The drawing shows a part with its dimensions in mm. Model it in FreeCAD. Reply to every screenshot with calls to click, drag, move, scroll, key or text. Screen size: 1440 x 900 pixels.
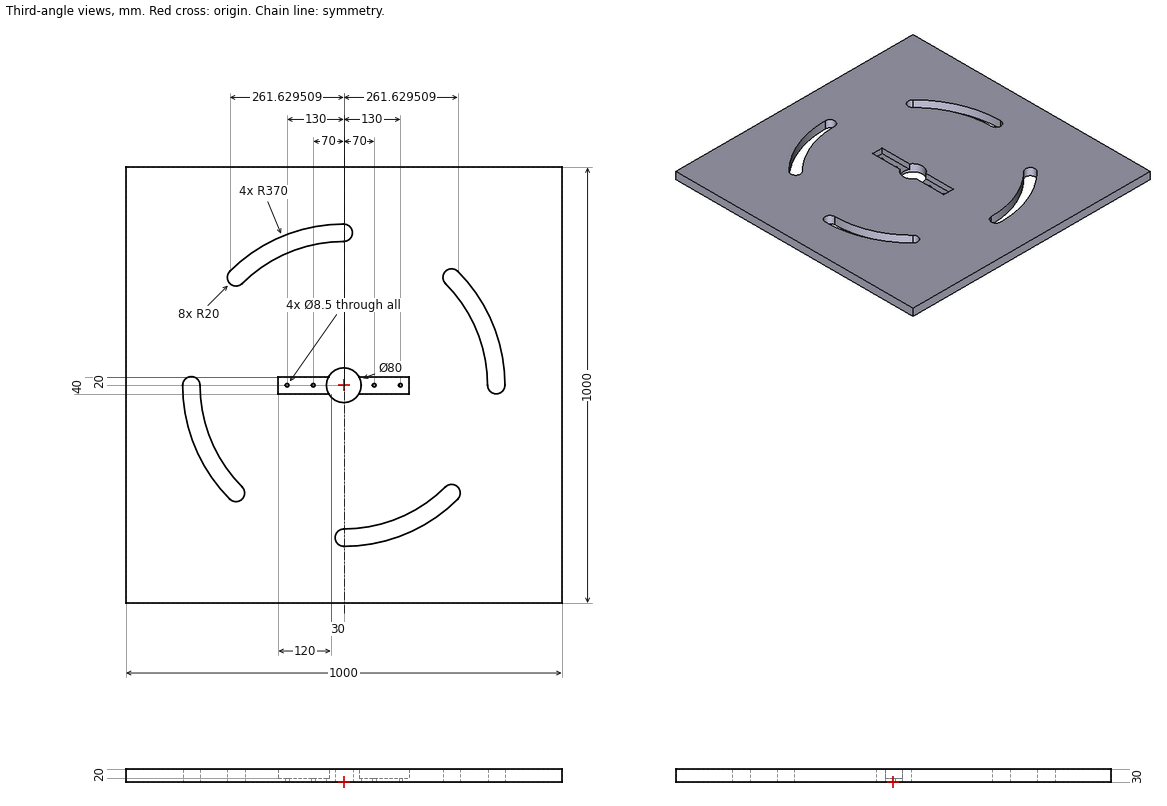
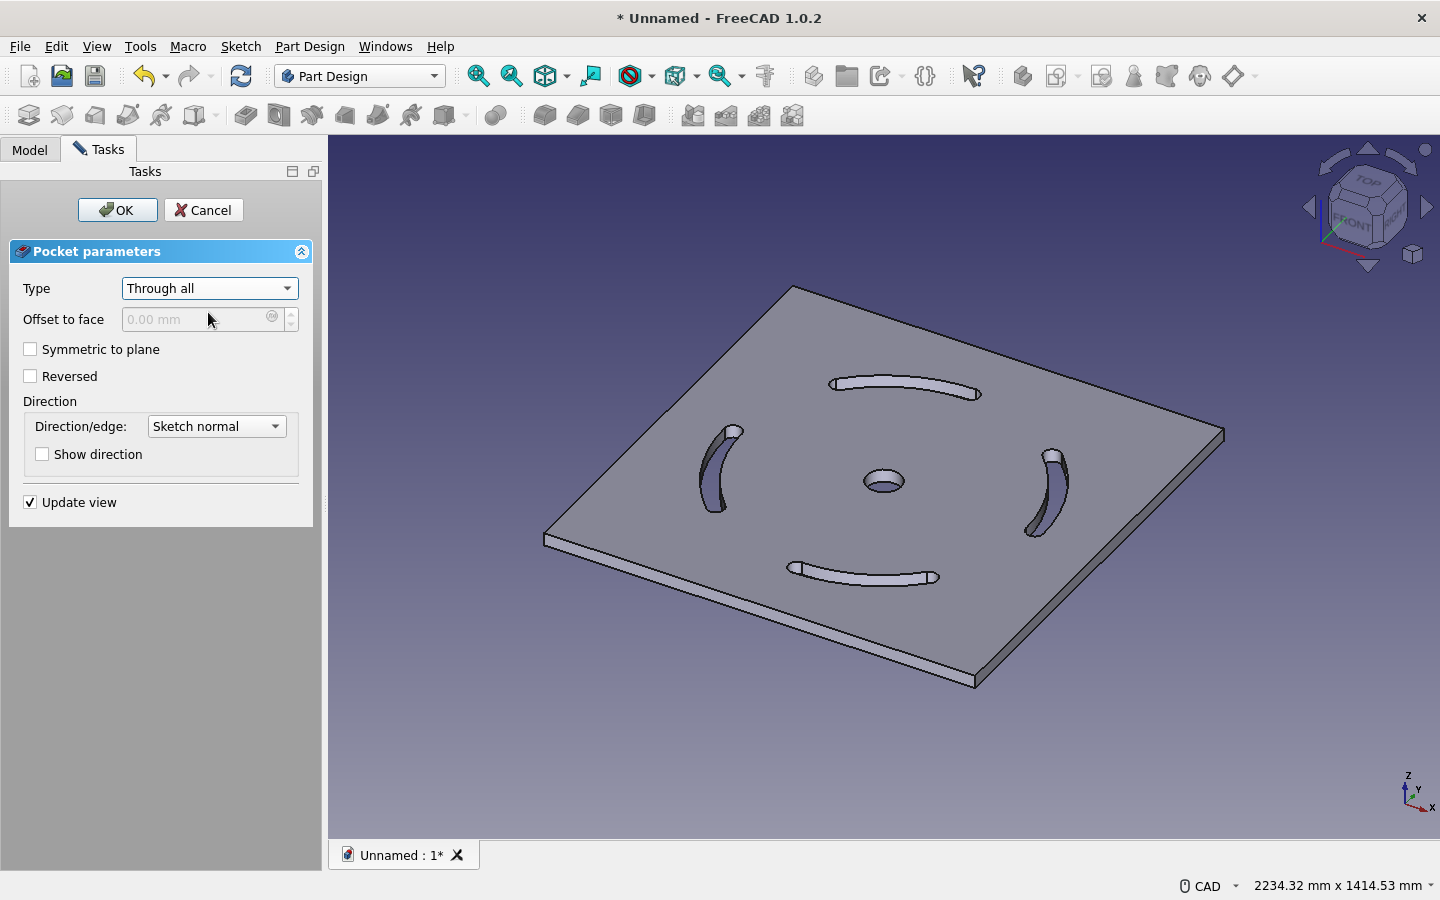
click(118, 210)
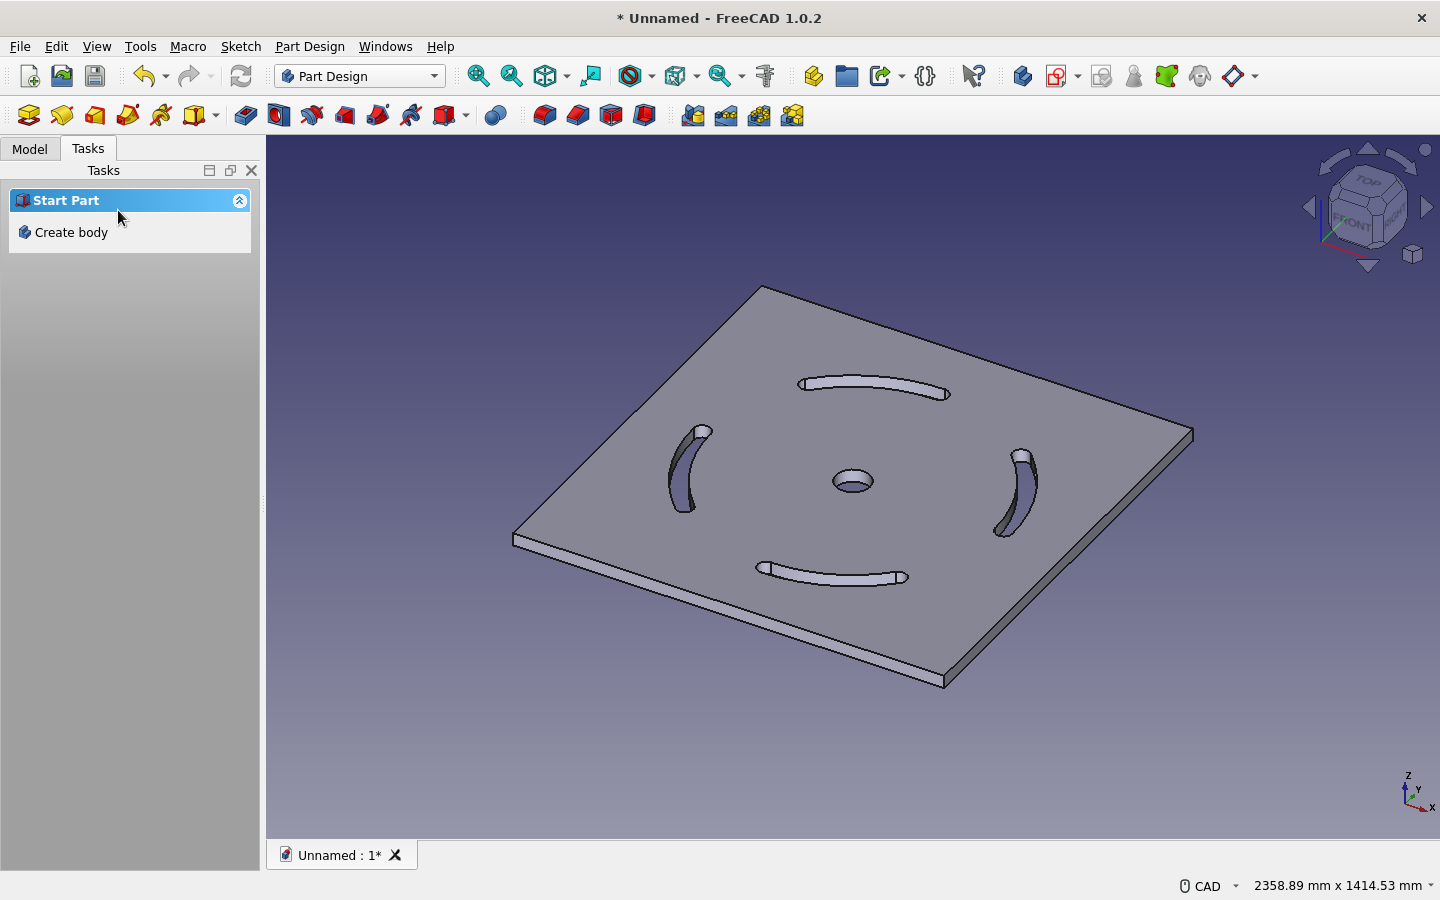
click(756, 495)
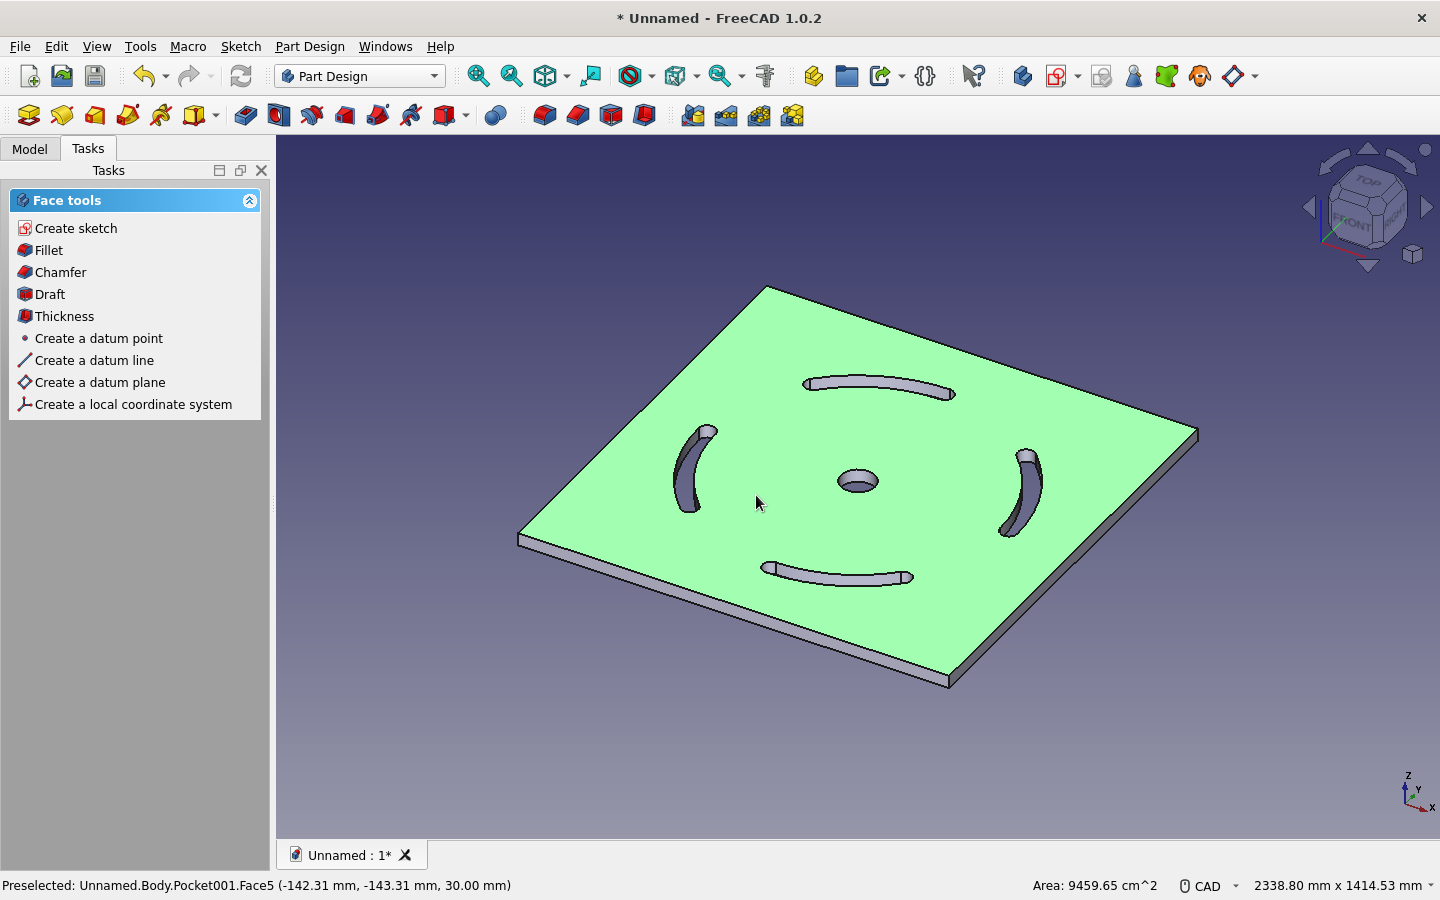
click(1056, 76)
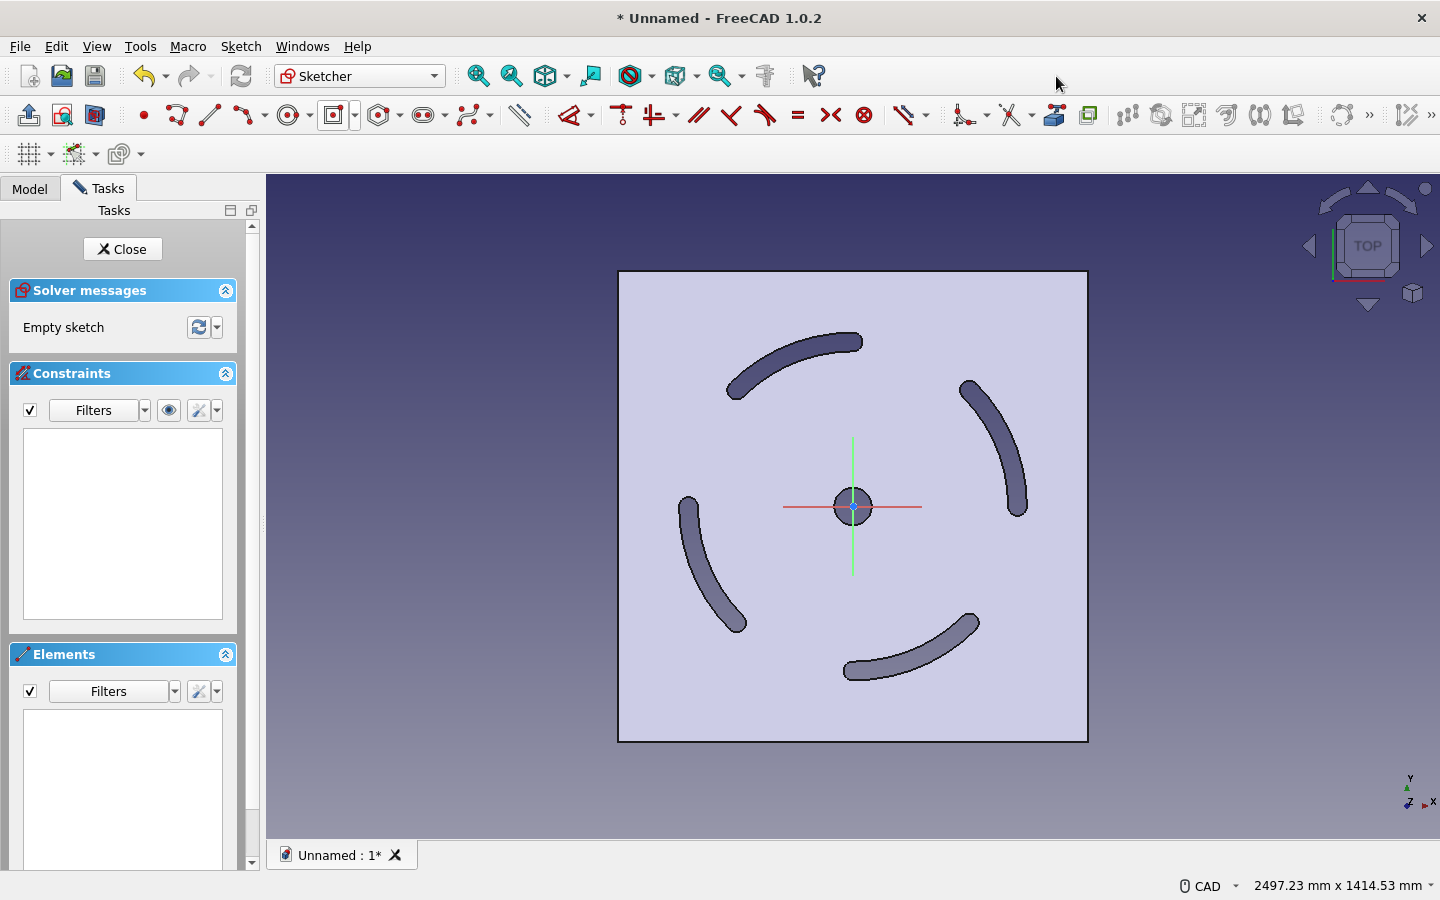
scroll(870, 506, up, 8)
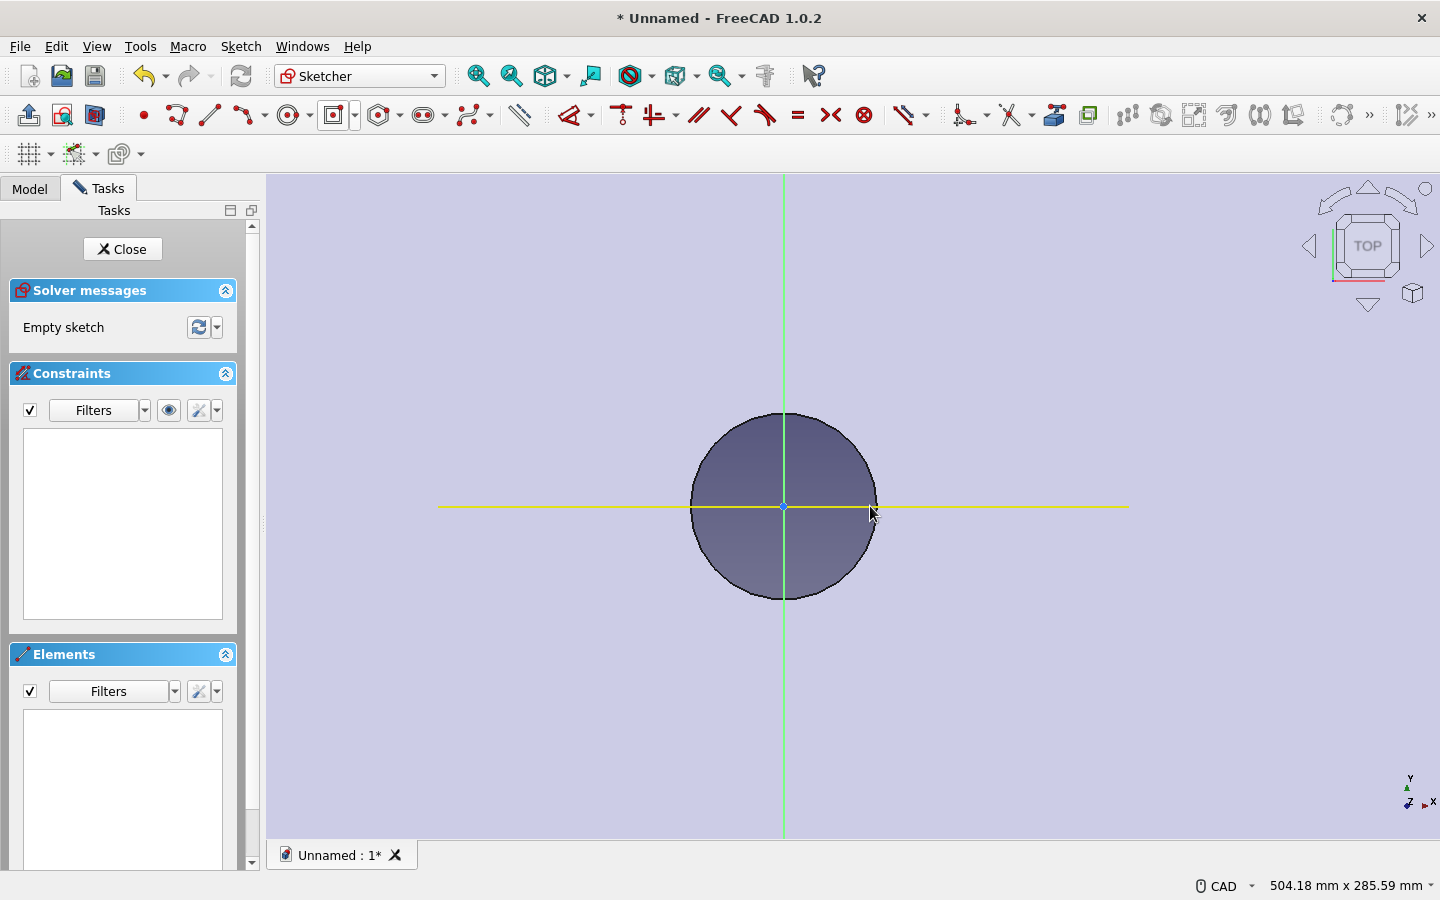
click(354, 116)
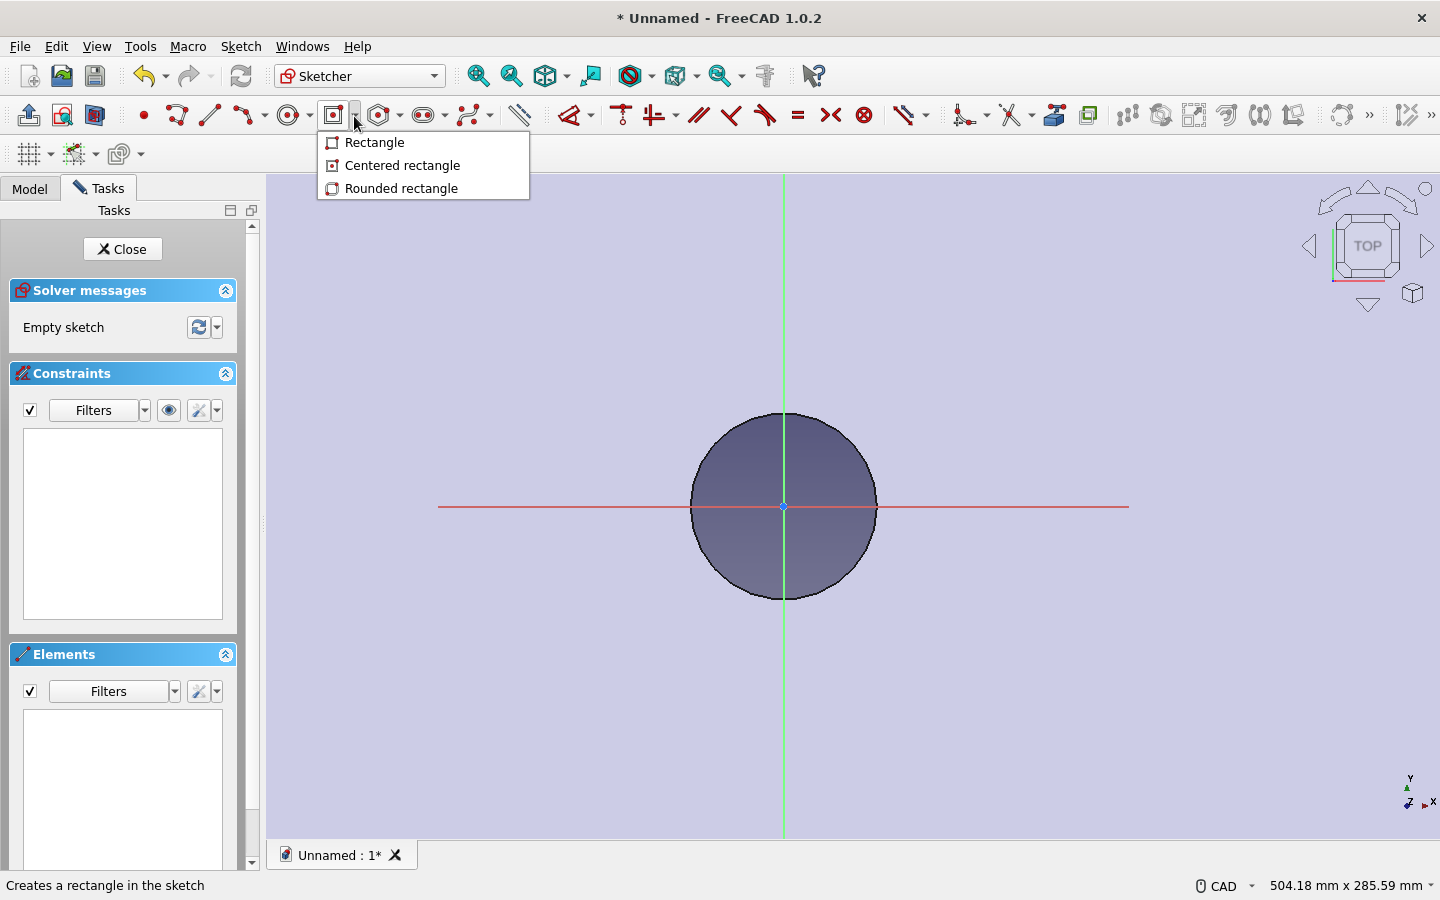
click(424, 142)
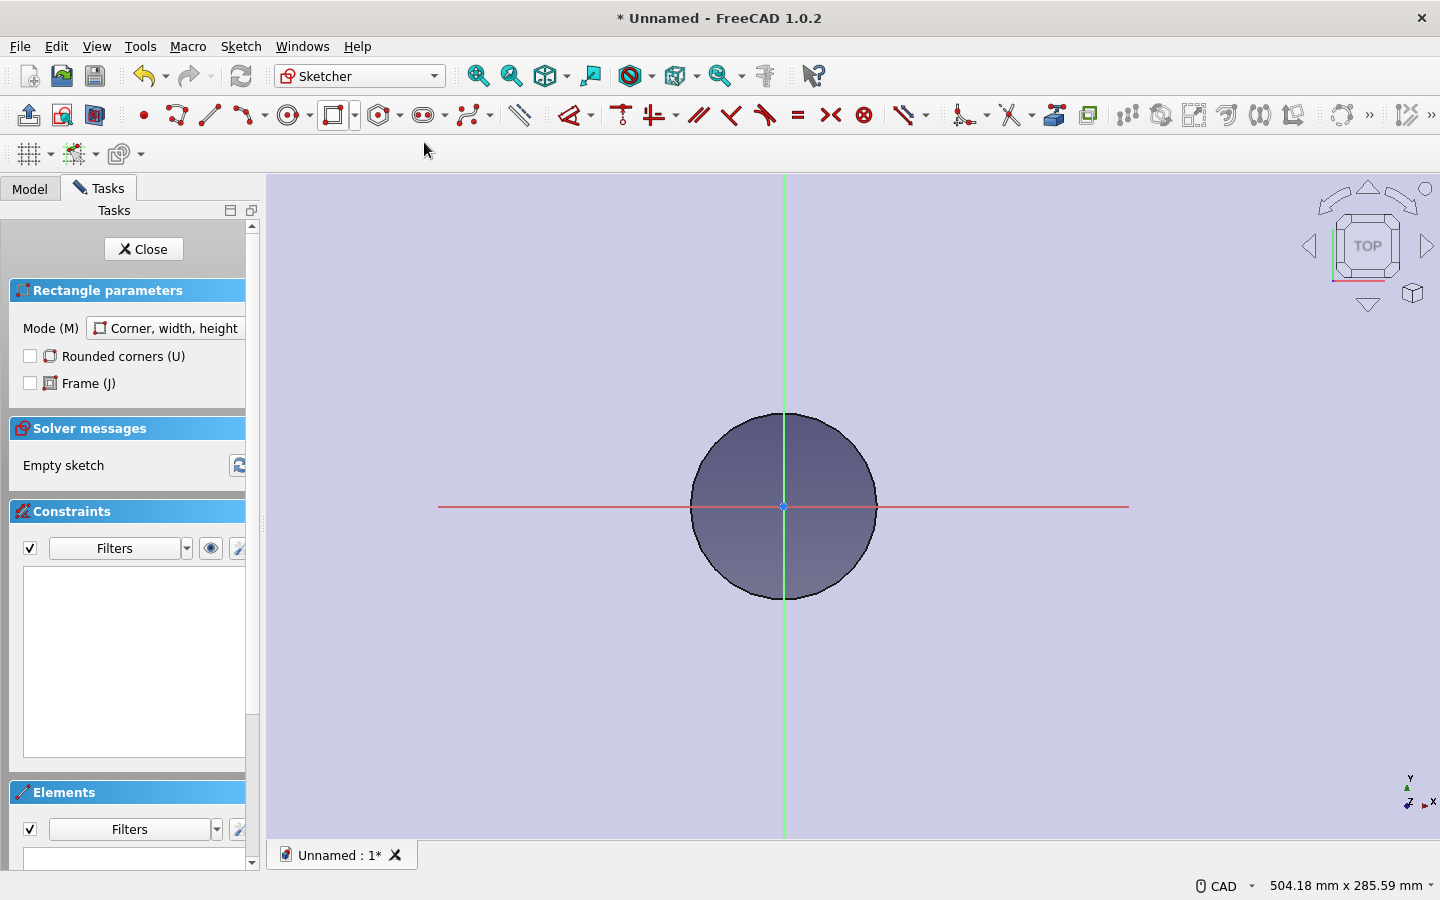
click(434, 460)
click(714, 553)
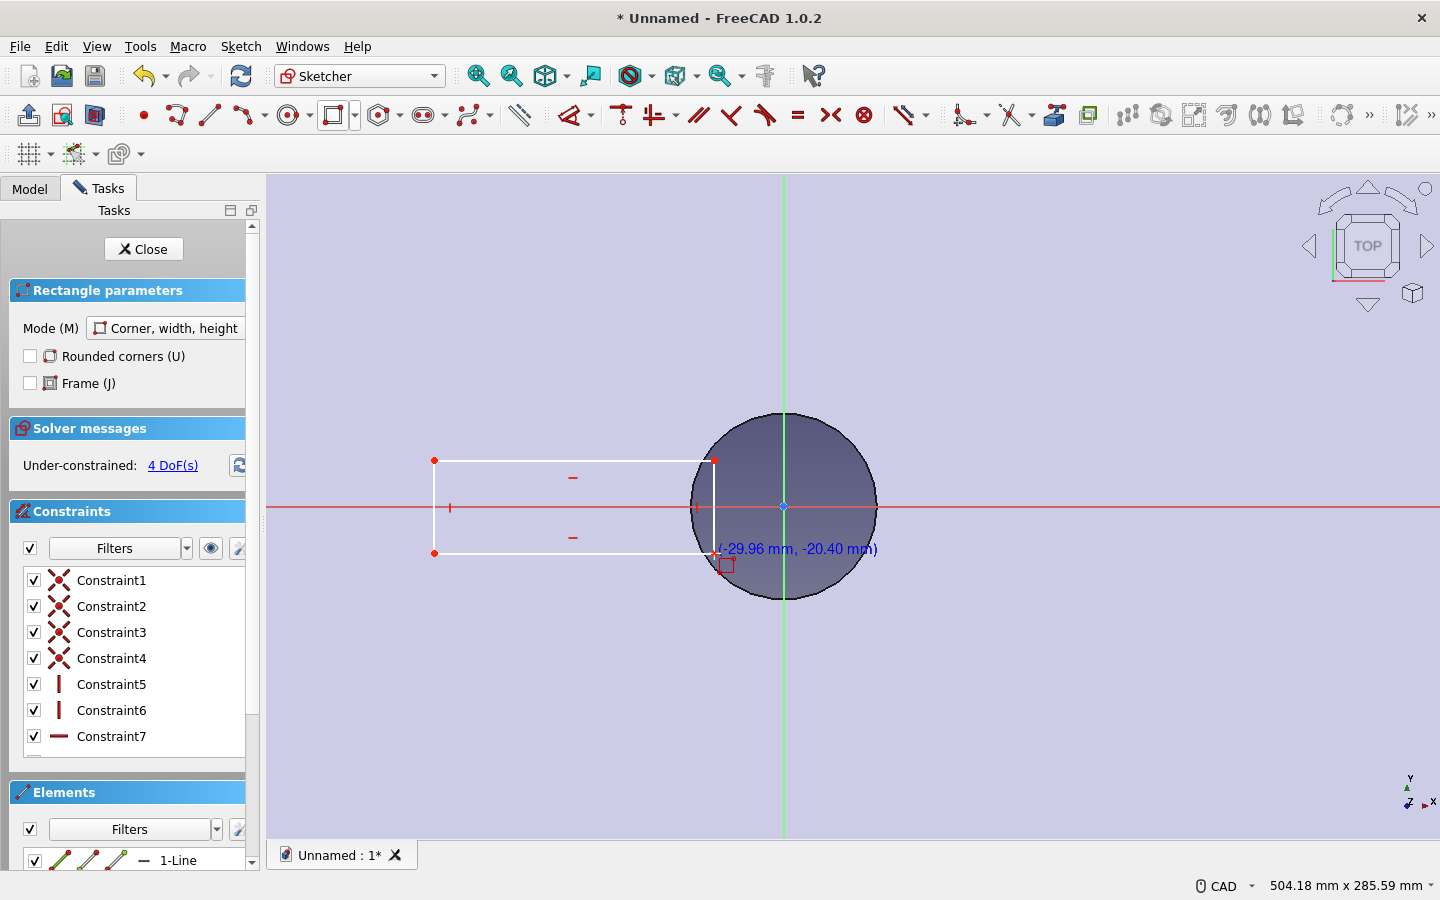
click(854, 460)
click(1133, 553)
key(Escape)